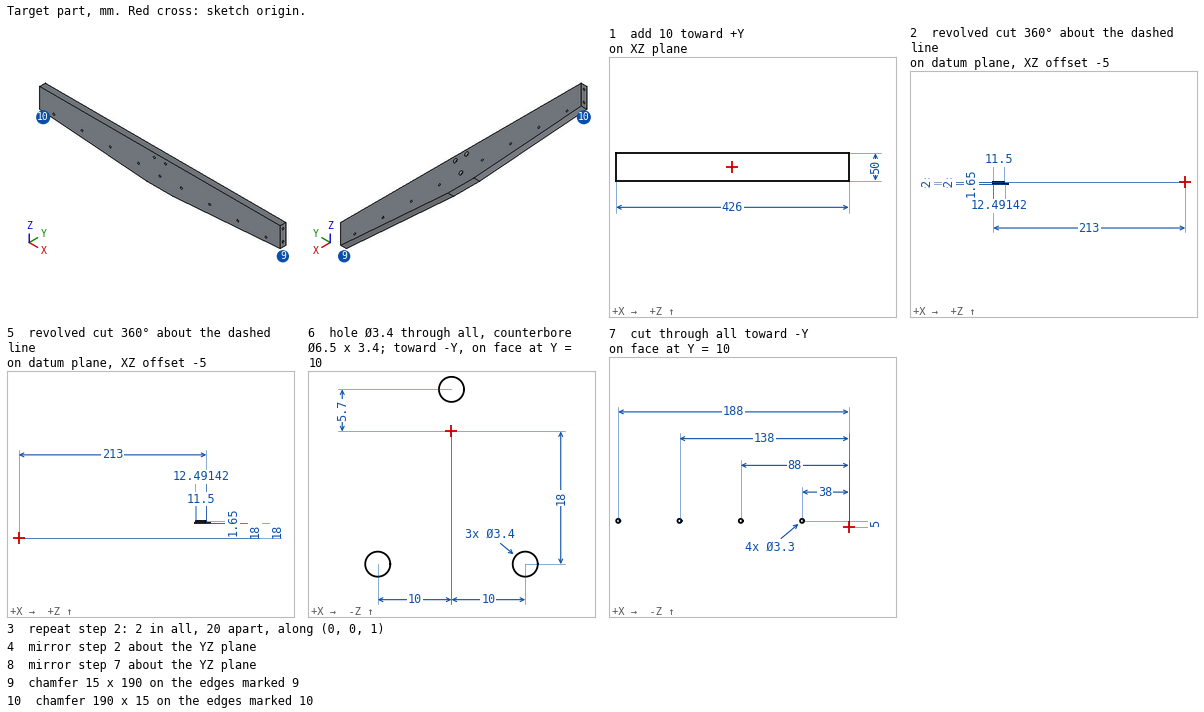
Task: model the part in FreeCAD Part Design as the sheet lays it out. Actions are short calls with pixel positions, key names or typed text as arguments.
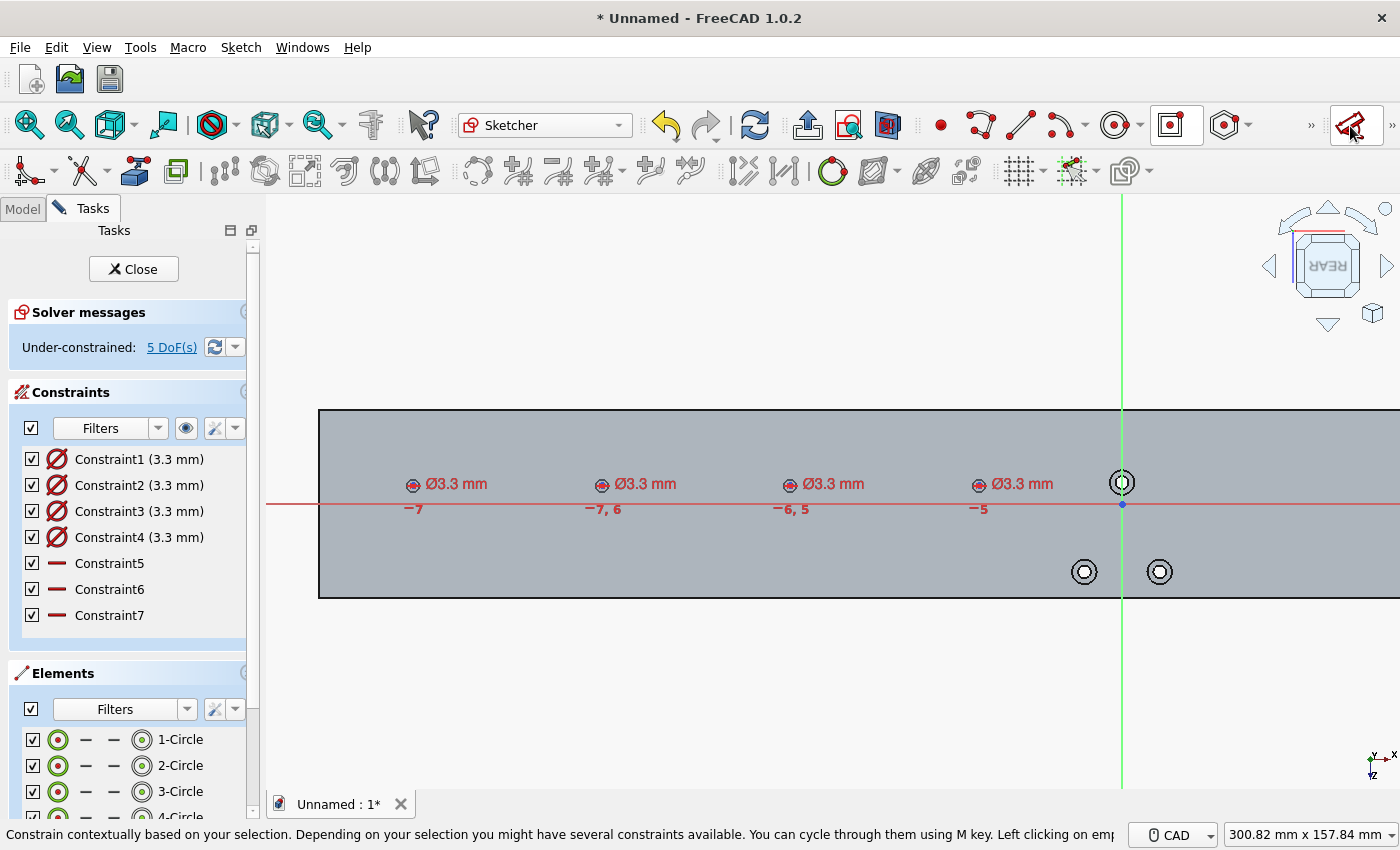
scroll(979, 486, up, 4)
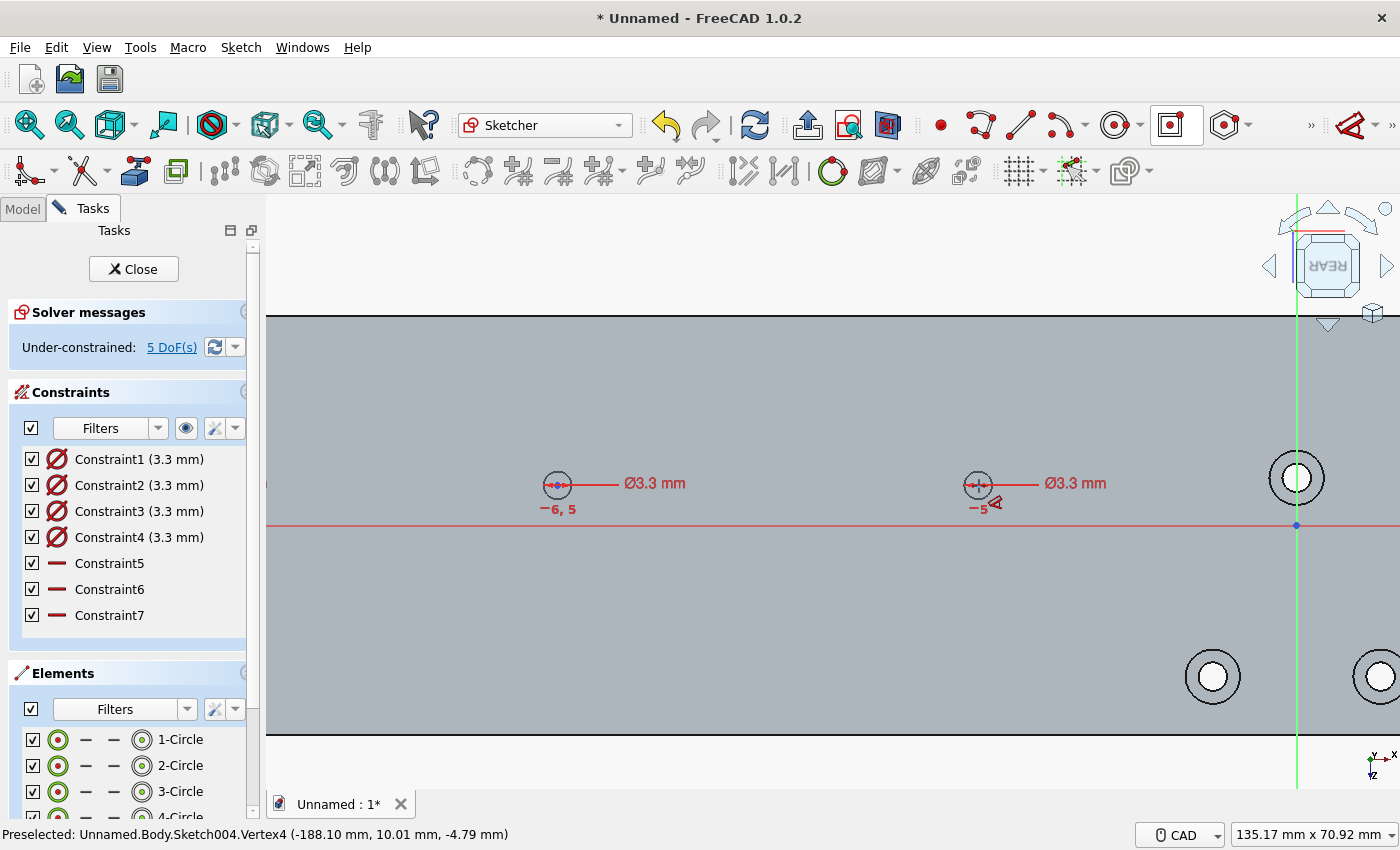
click(978, 485)
click(944, 506)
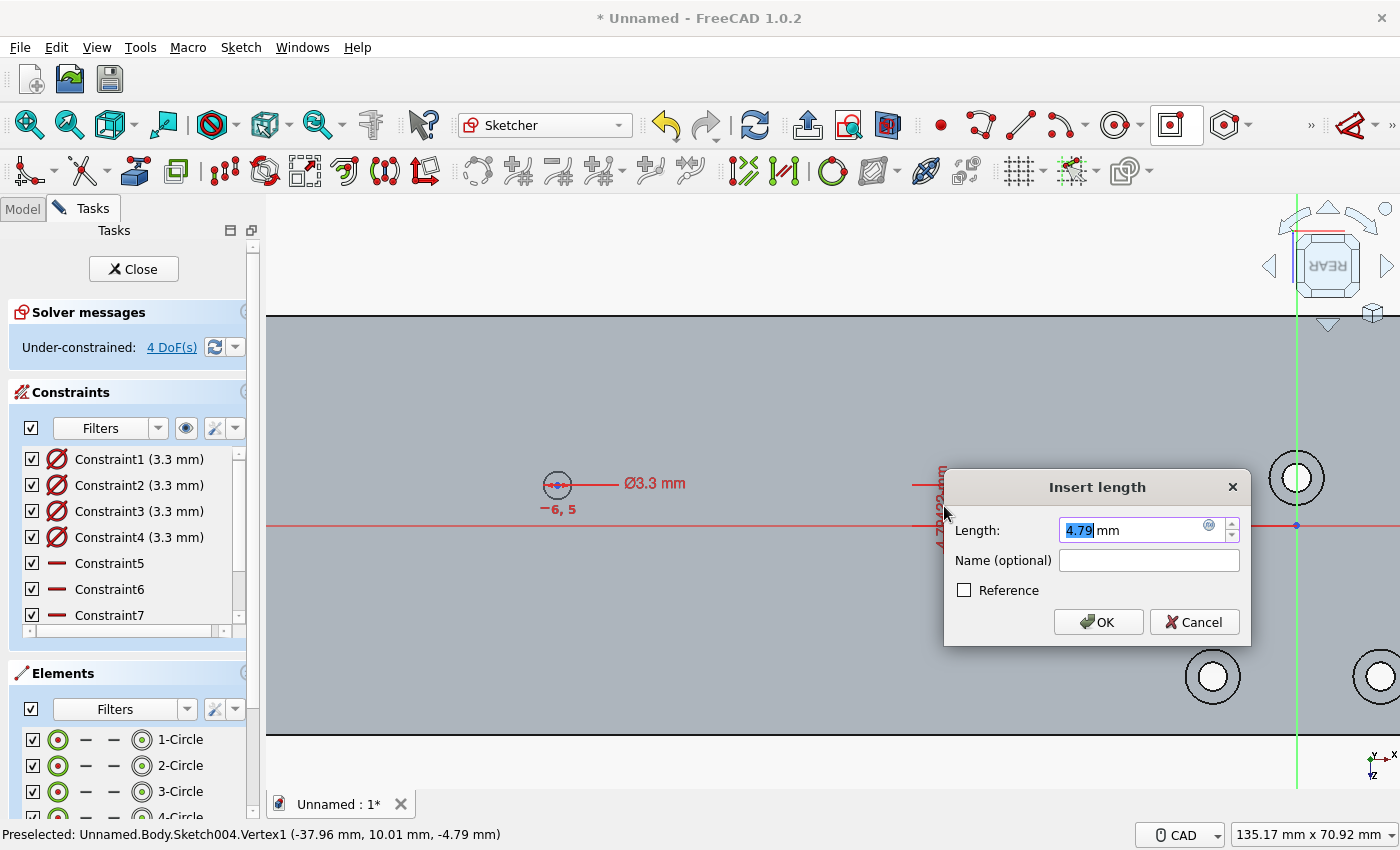
text(5)
key(Return)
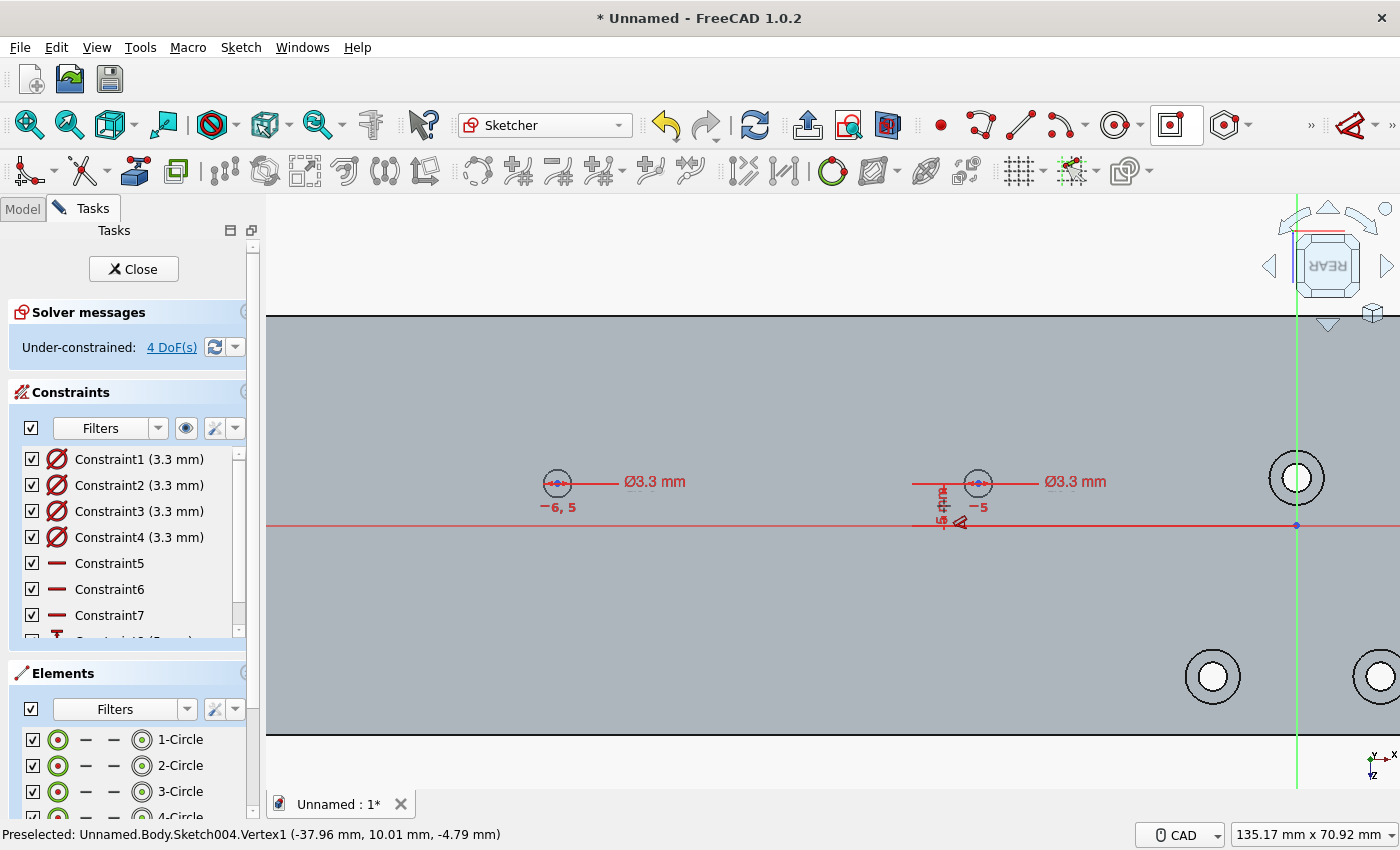
click(978, 484)
click(1107, 560)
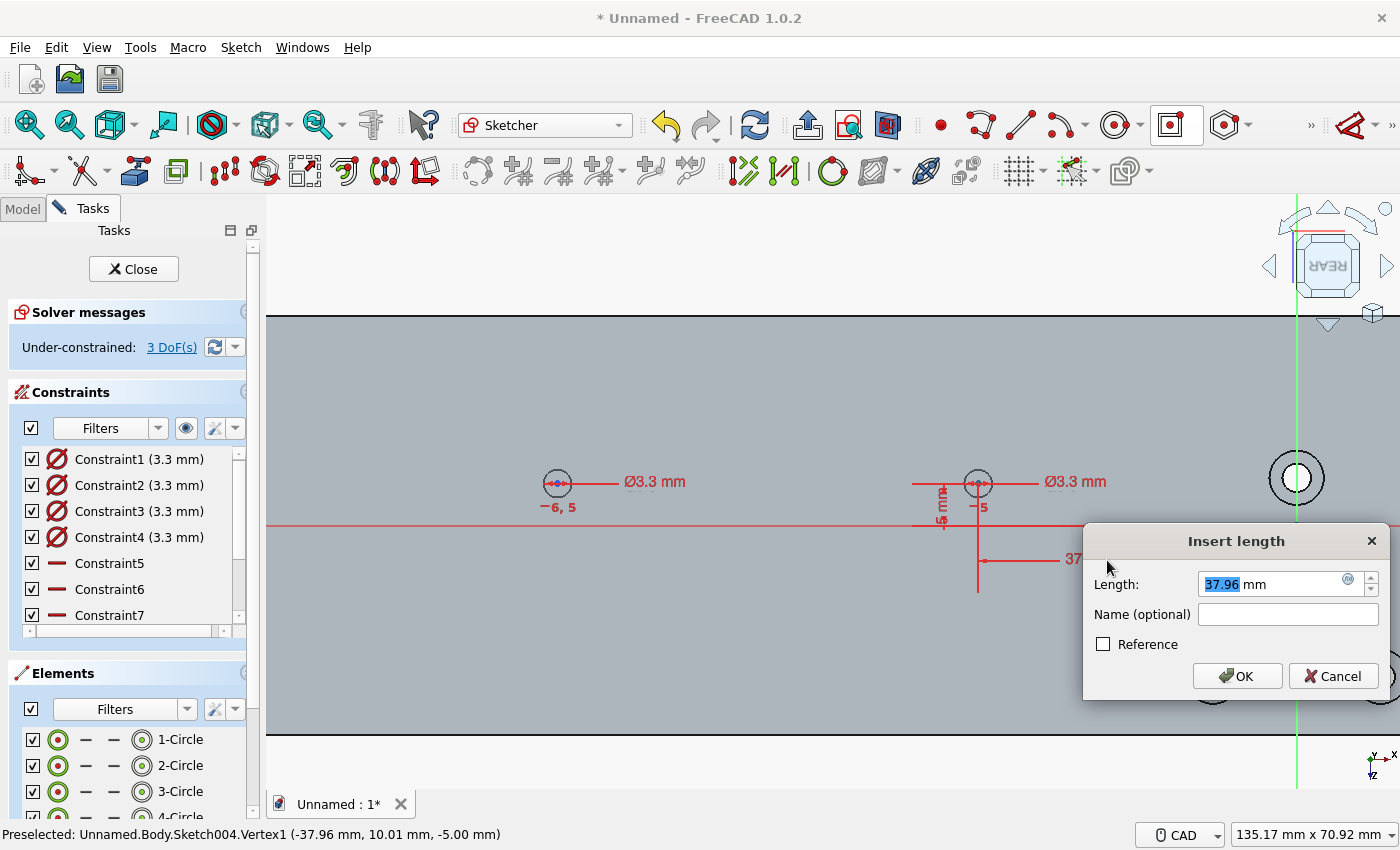
text(38)
key(Return)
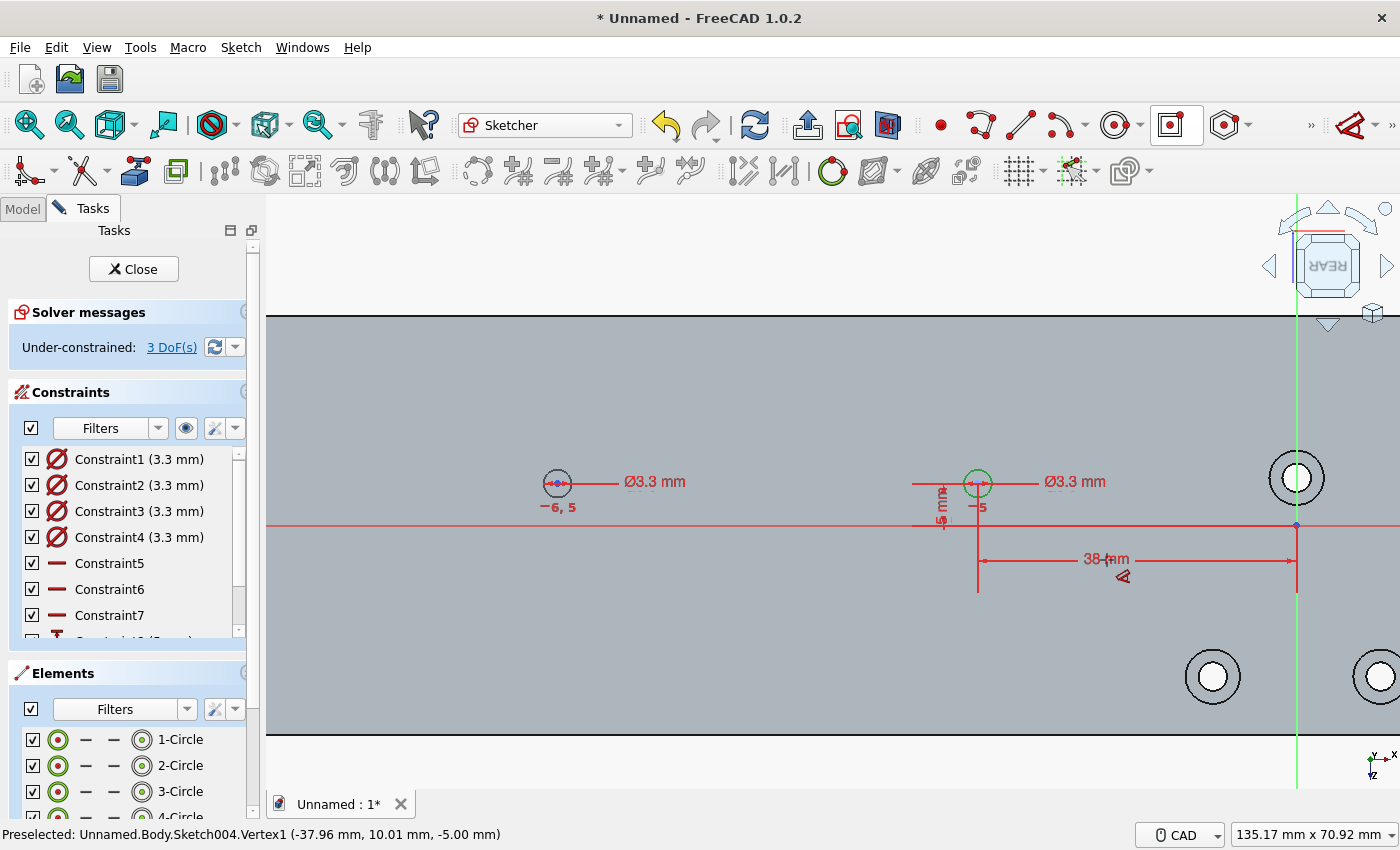
click(558, 484)
click(896, 560)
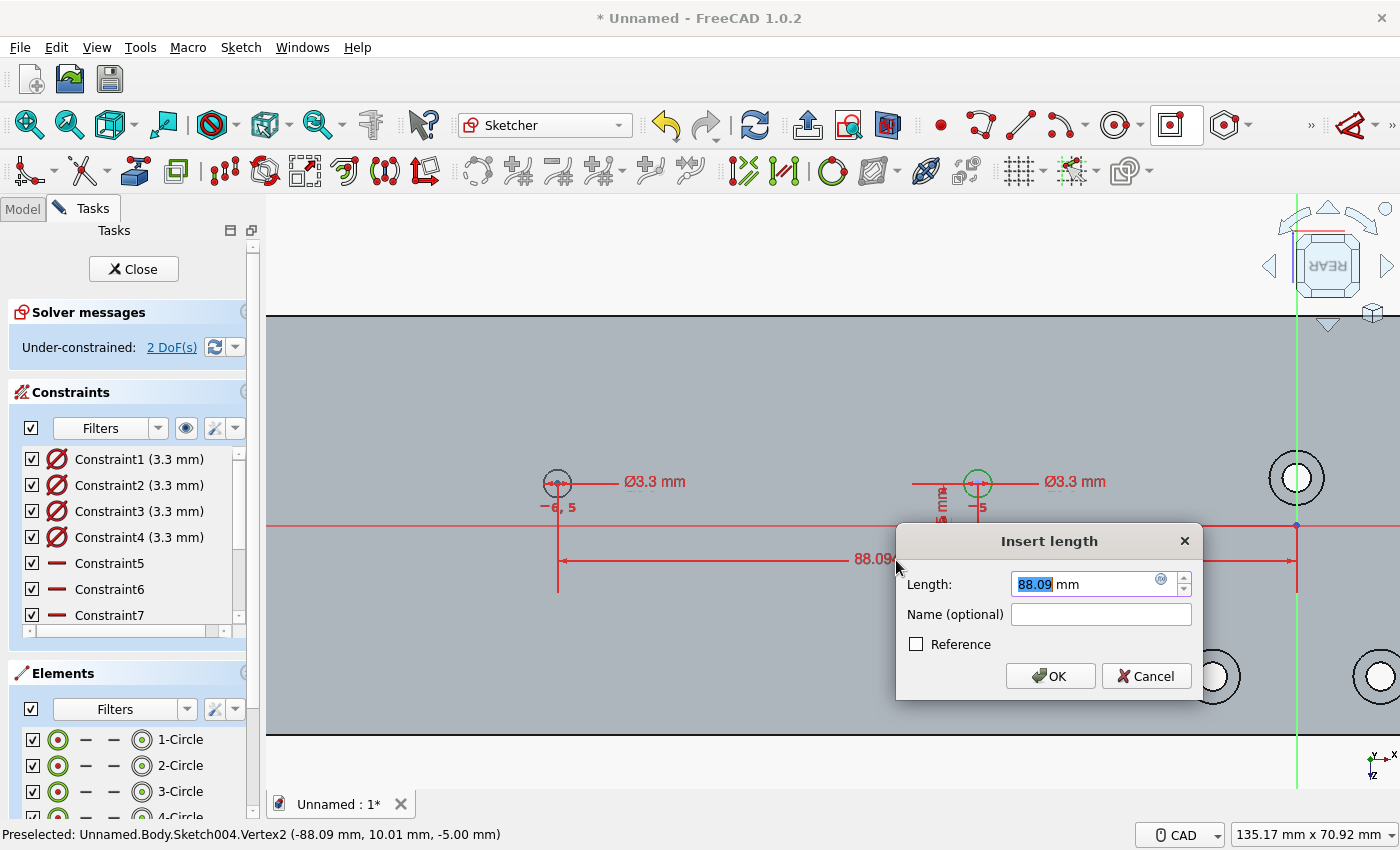
text(88)
key(Return)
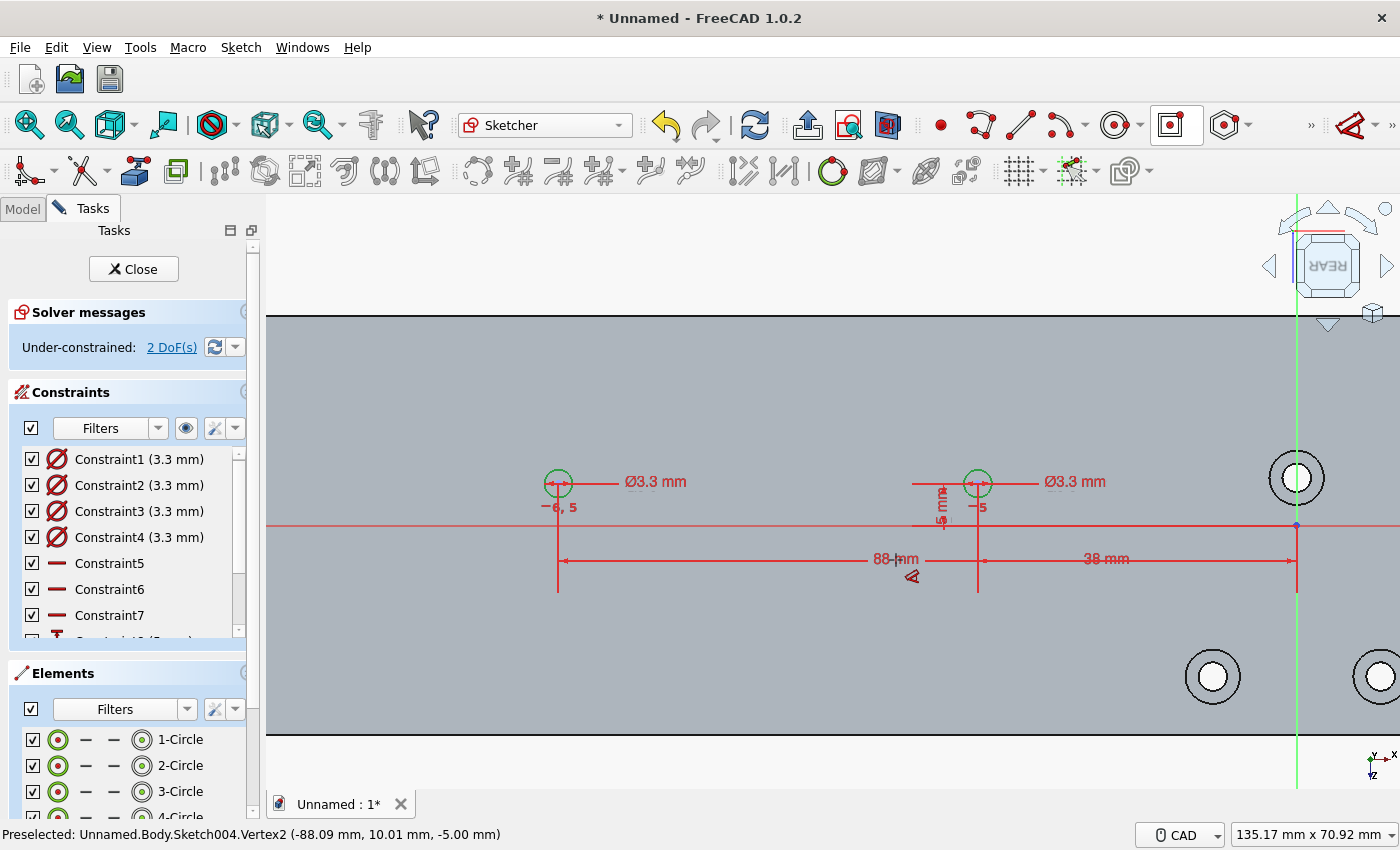
scroll(979, 486, down, 4)